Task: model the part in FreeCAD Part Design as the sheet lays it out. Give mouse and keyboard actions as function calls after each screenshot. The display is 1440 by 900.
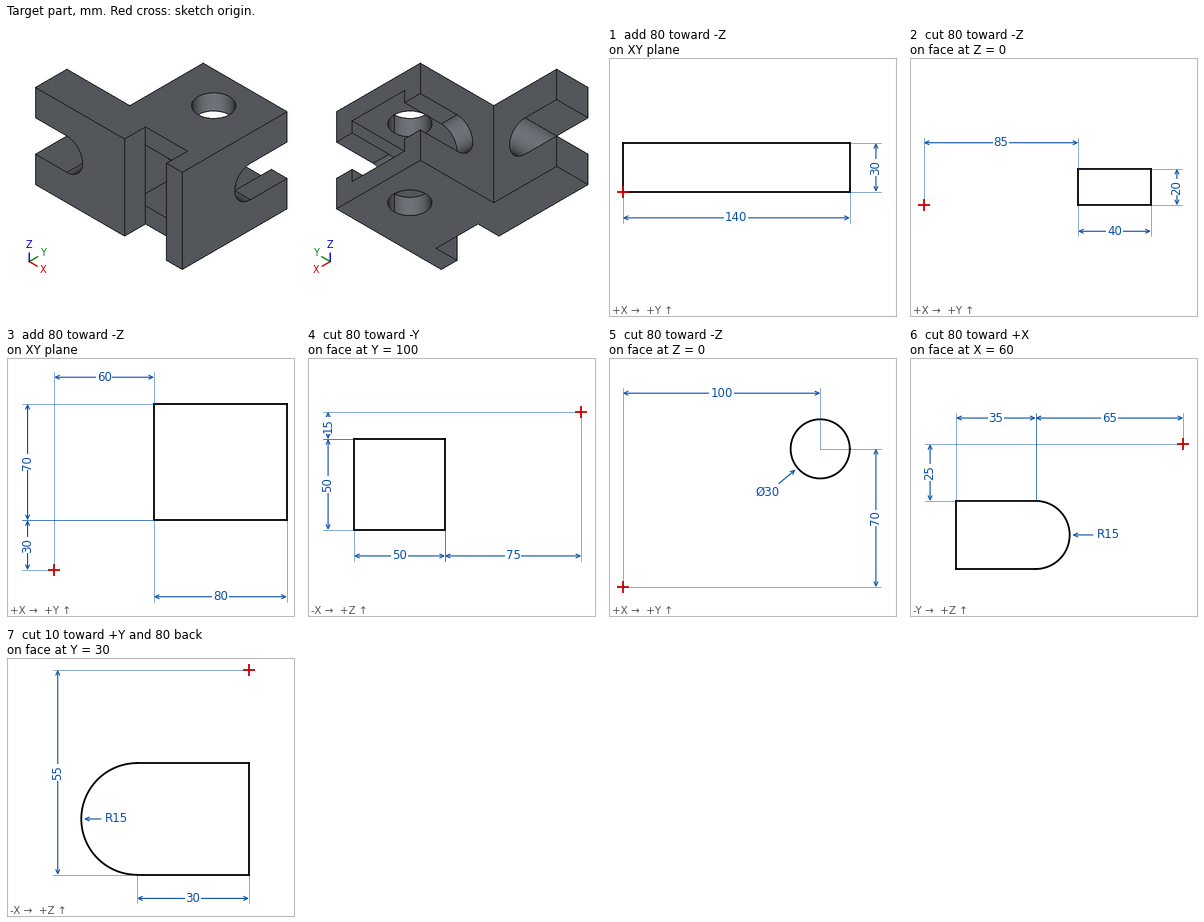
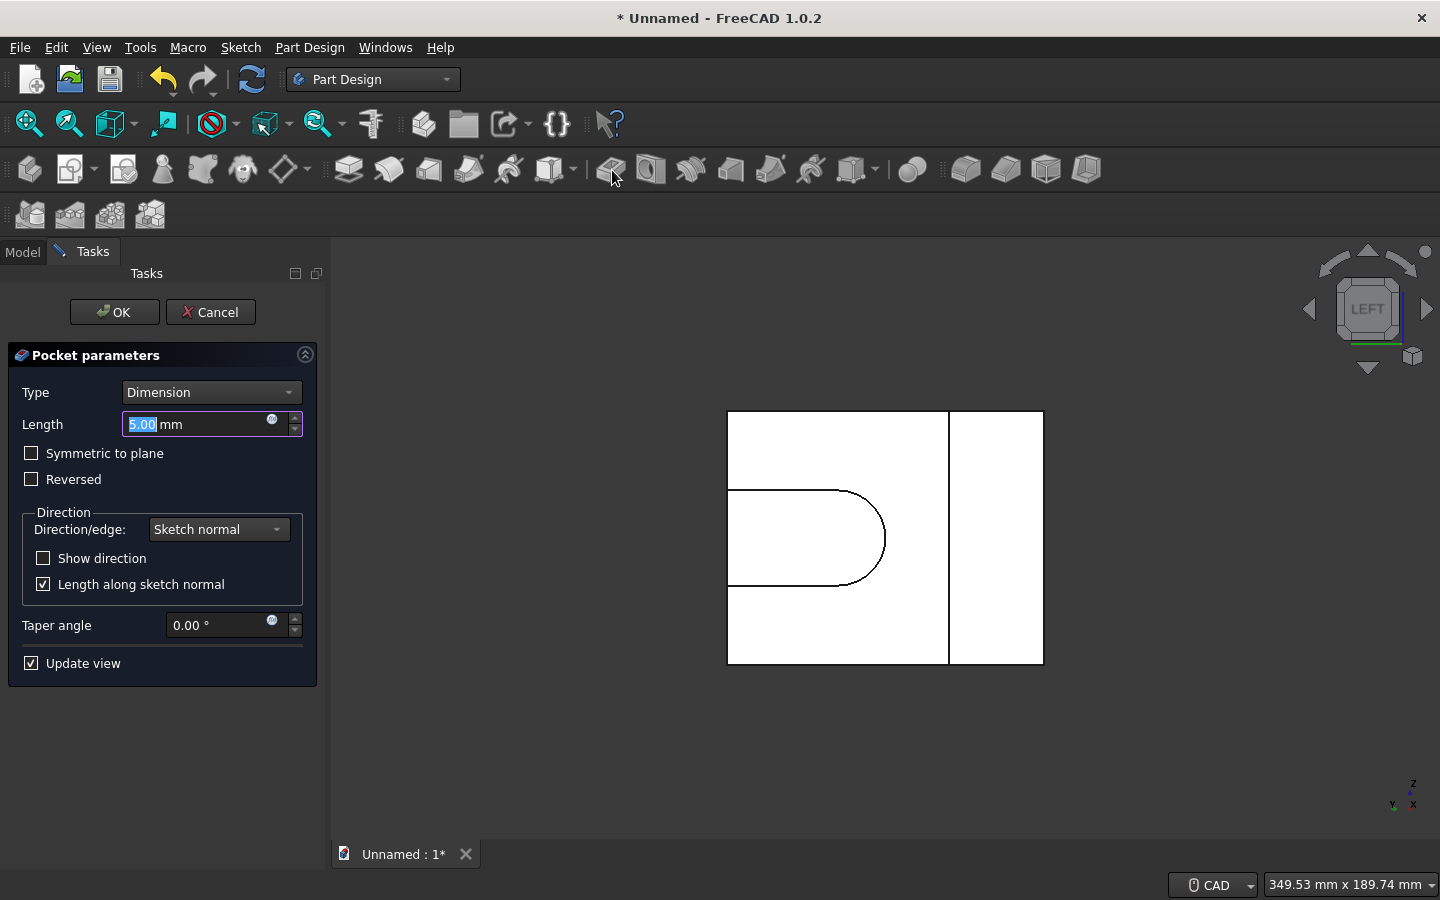
text(80)
key(Tab)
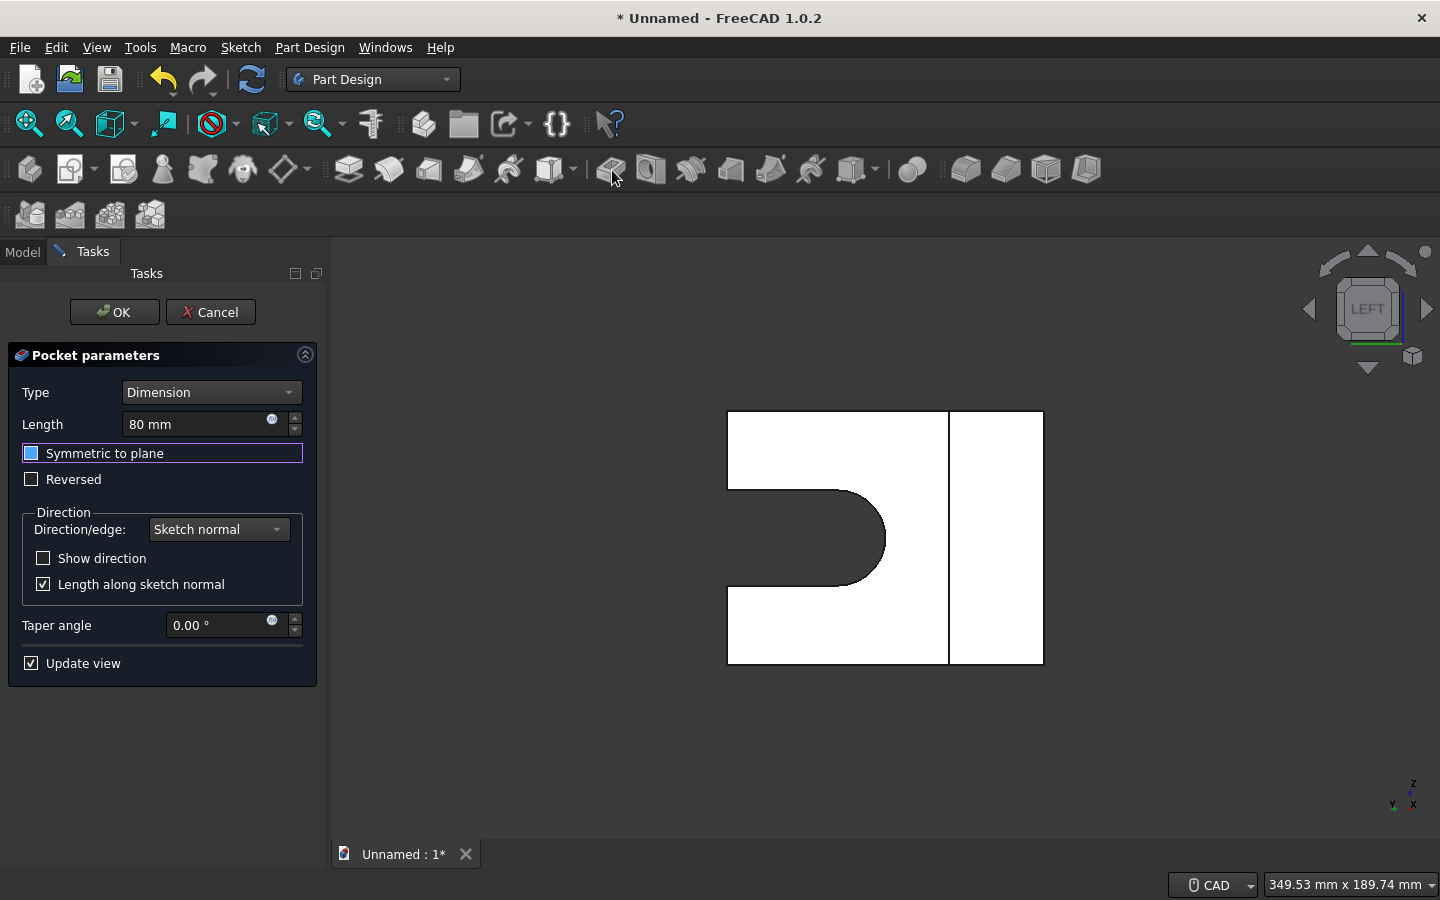
click(115, 312)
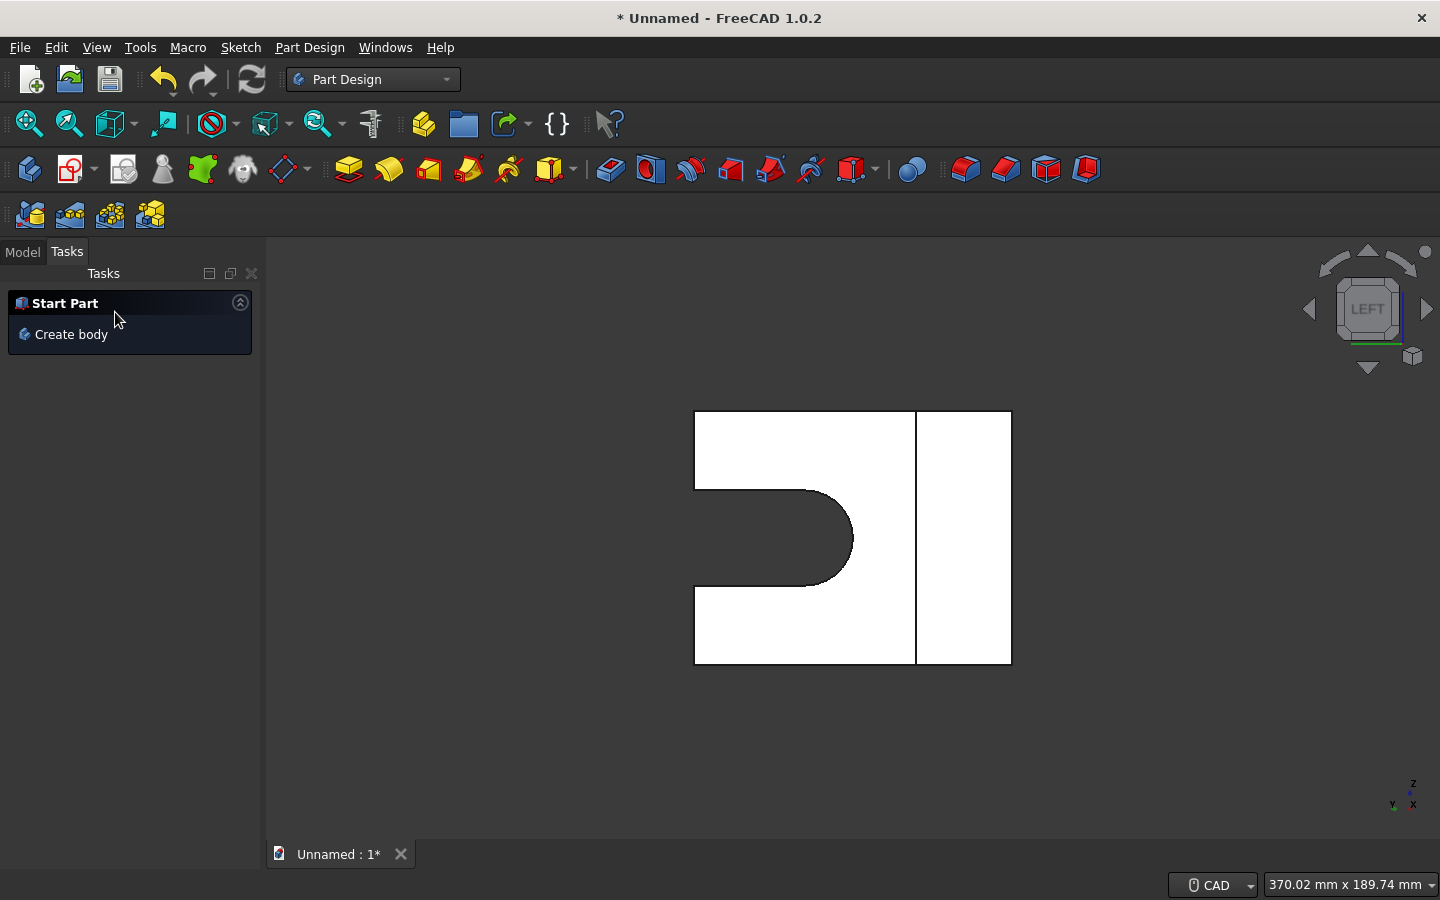
click(30, 124)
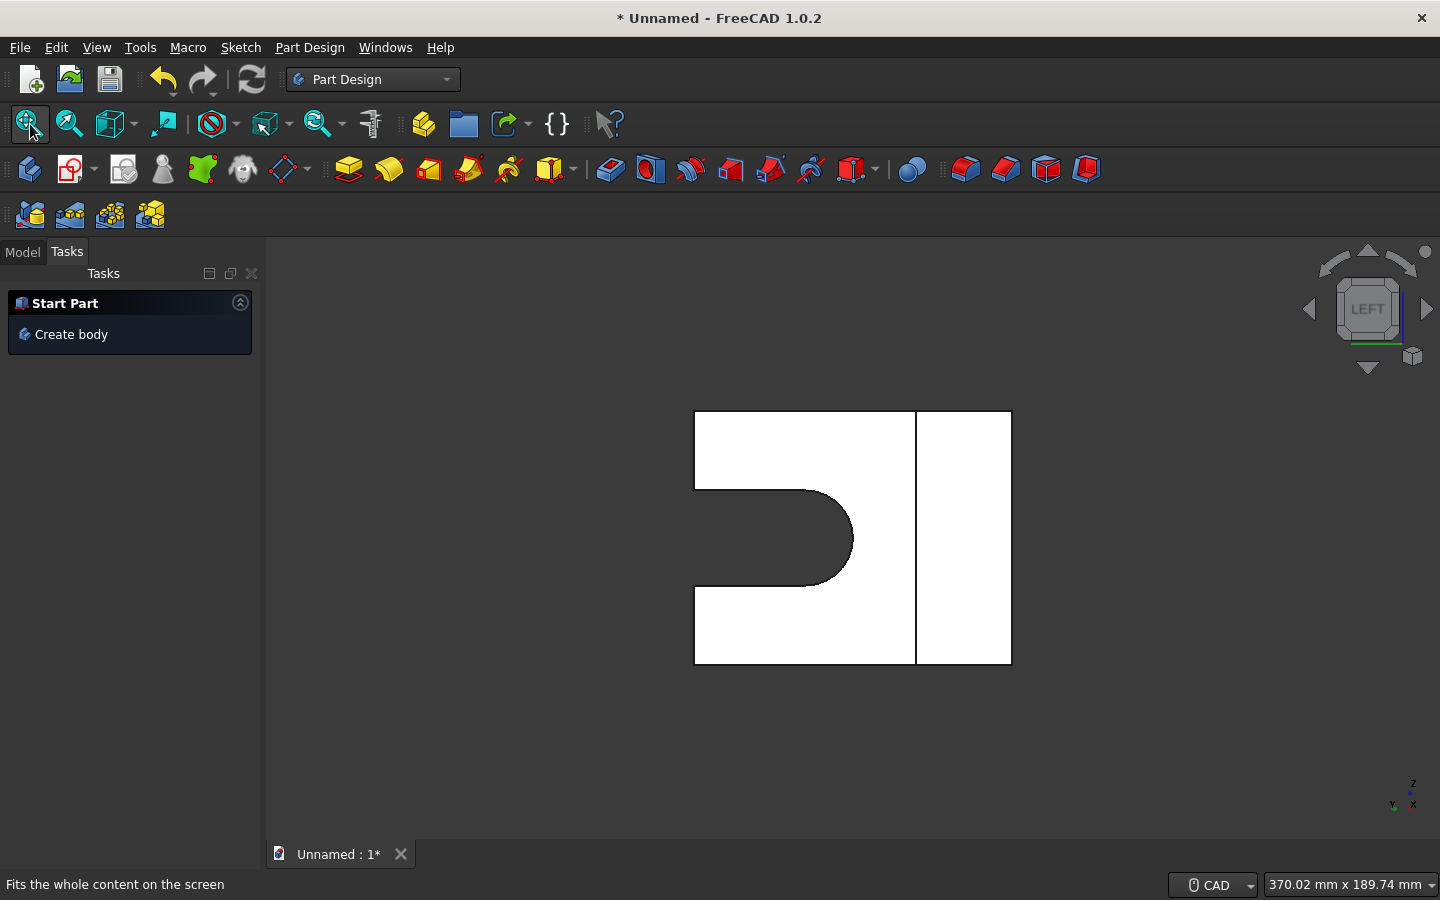
key(4)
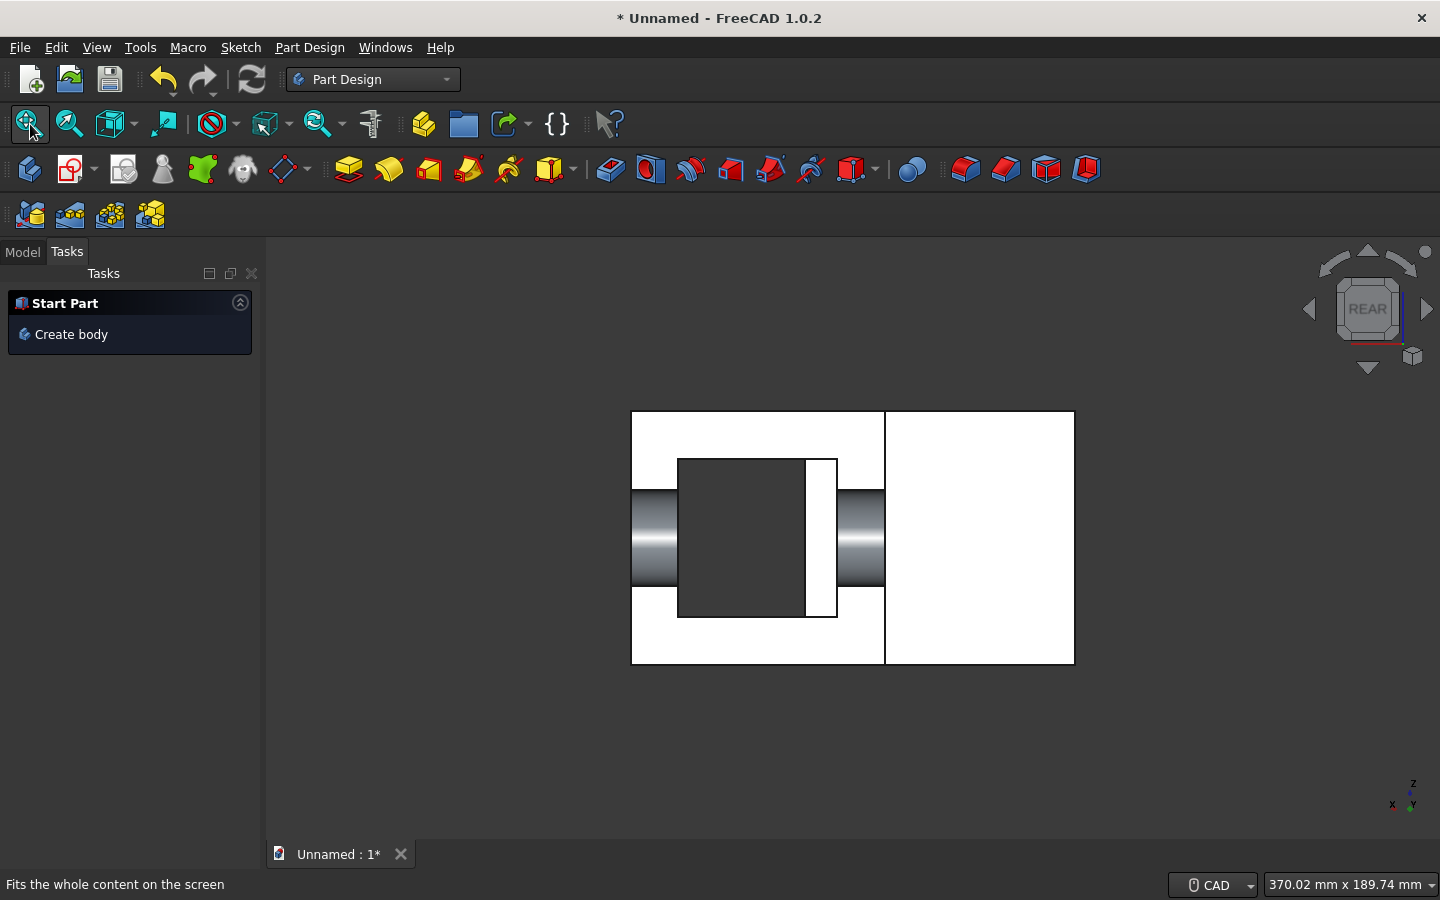
key(v)
key(f)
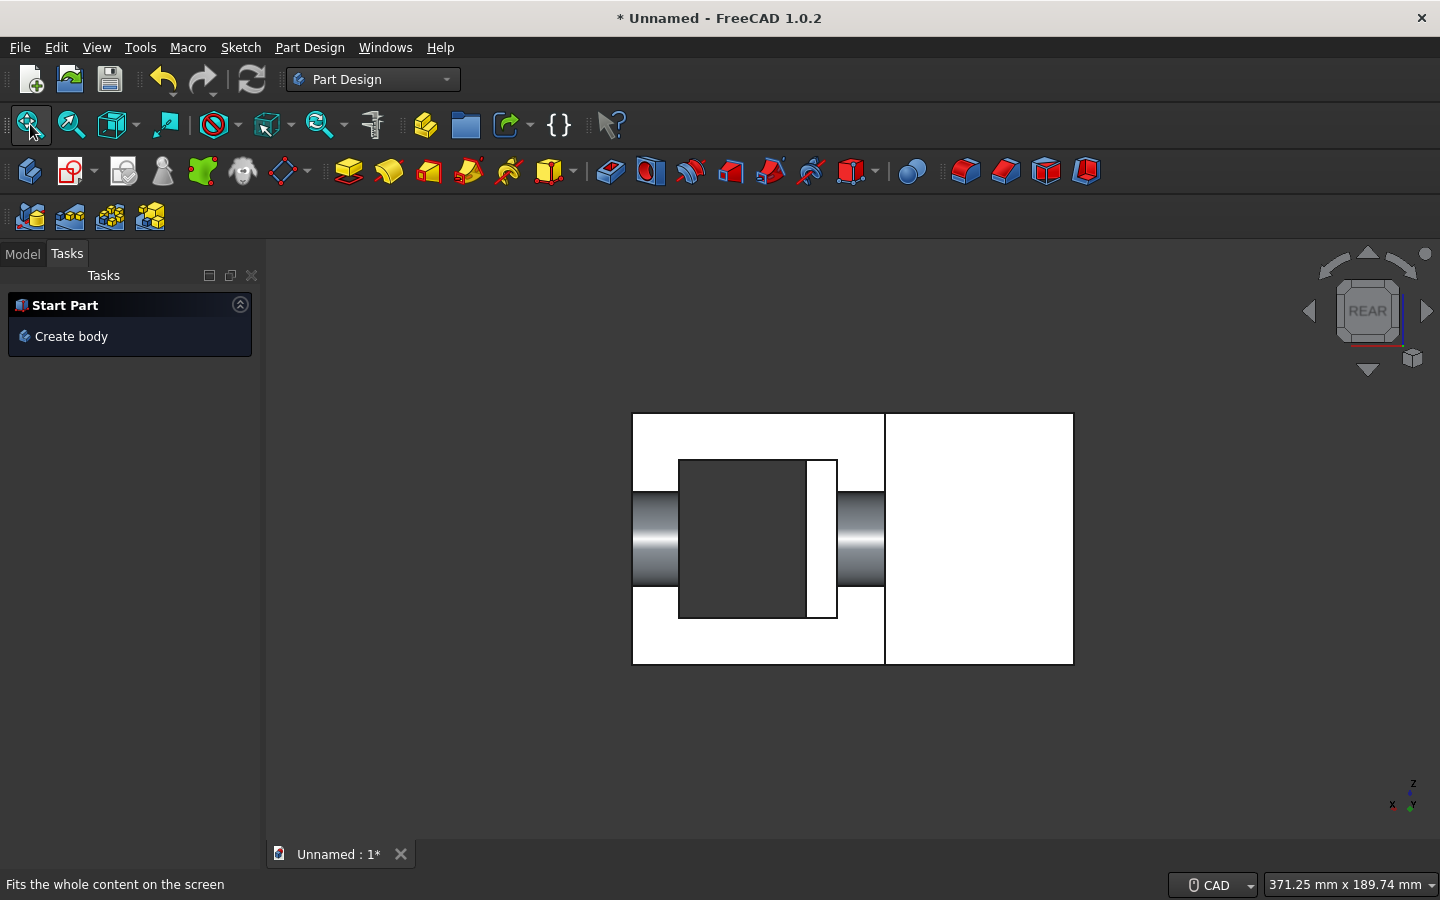
click(979, 538)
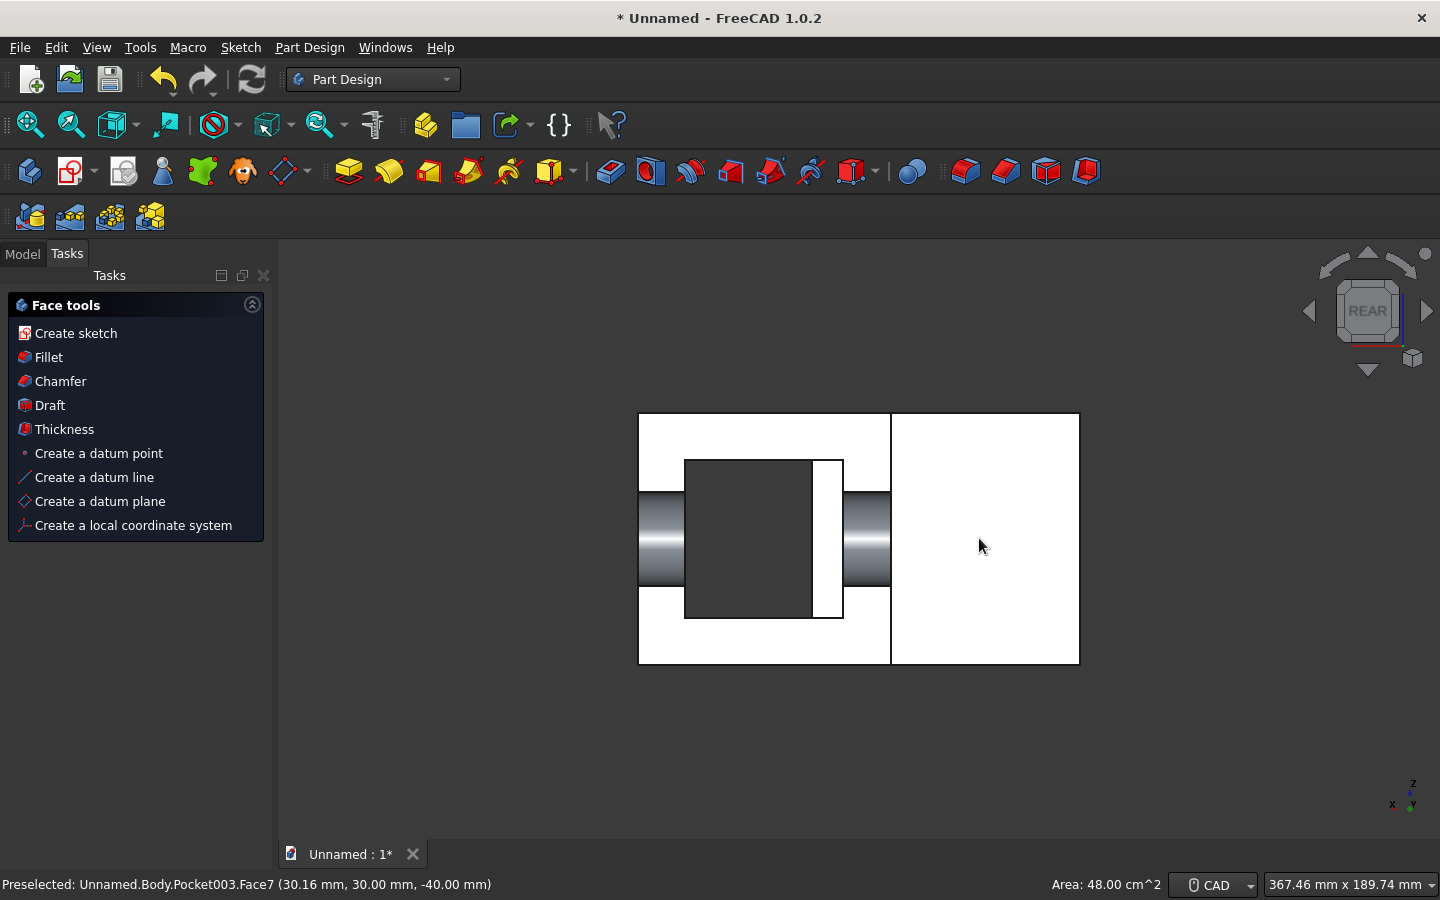
click(70, 172)